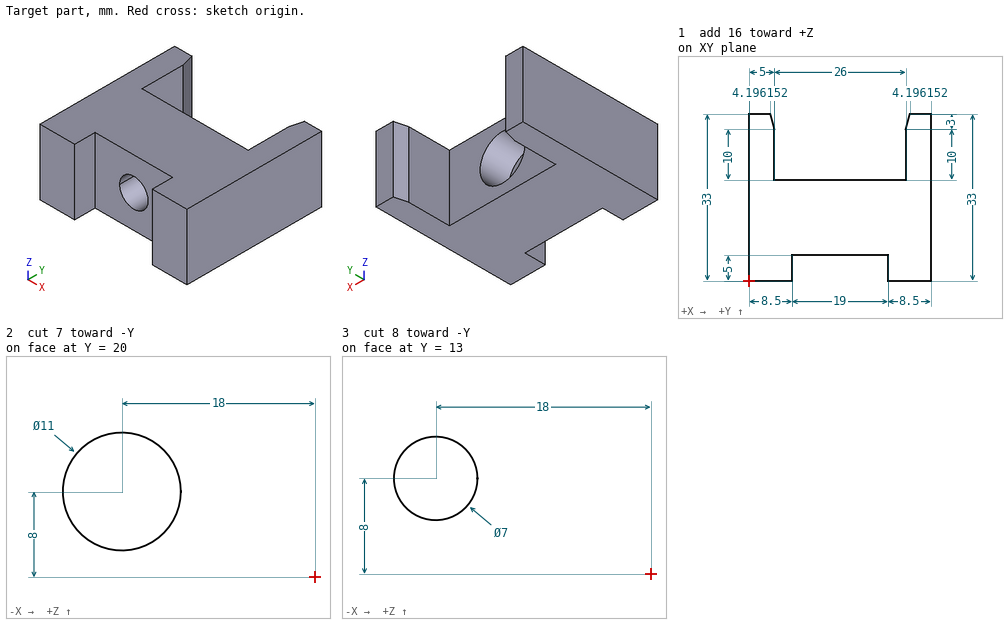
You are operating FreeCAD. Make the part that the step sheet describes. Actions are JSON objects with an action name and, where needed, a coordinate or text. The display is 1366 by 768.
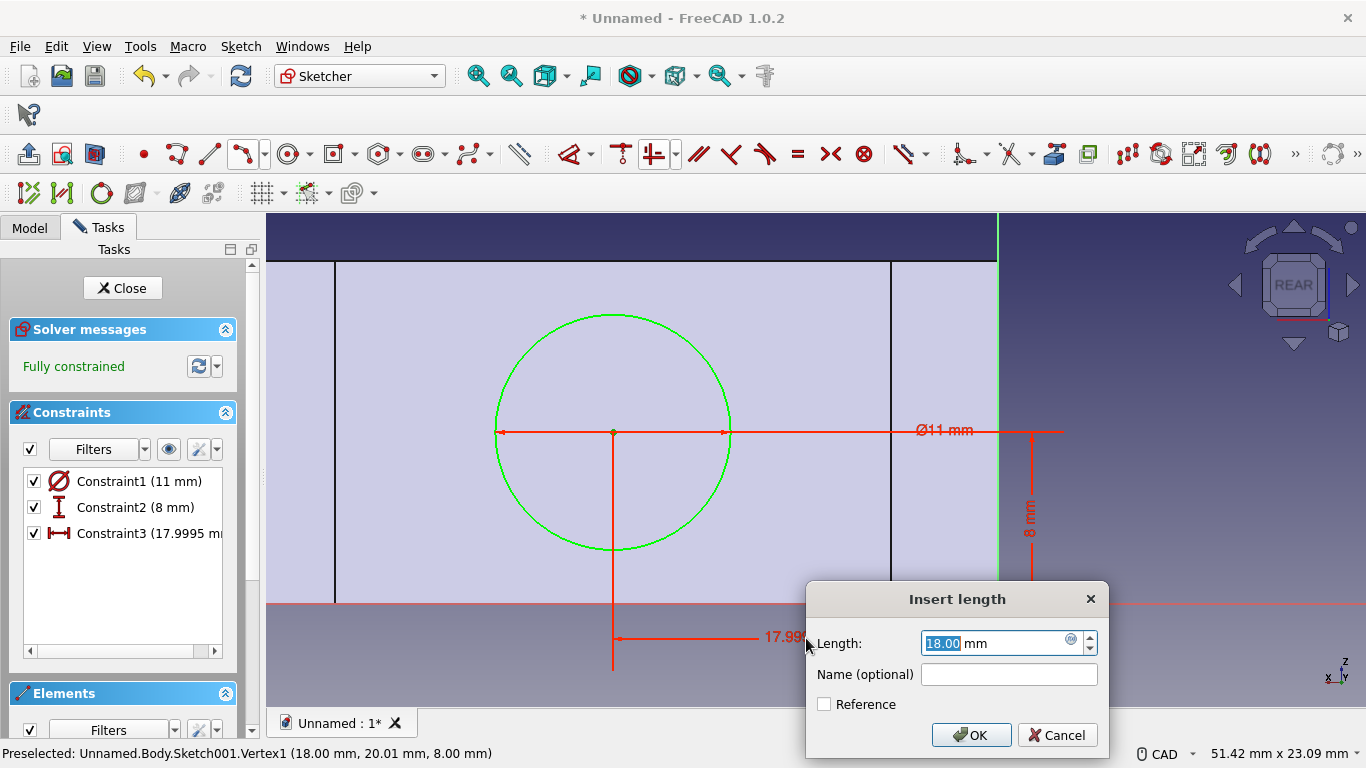
{"action": "type", "text": "18"}
{"action": "key", "text": "Return"}
{"action": "key", "text": "Escape"}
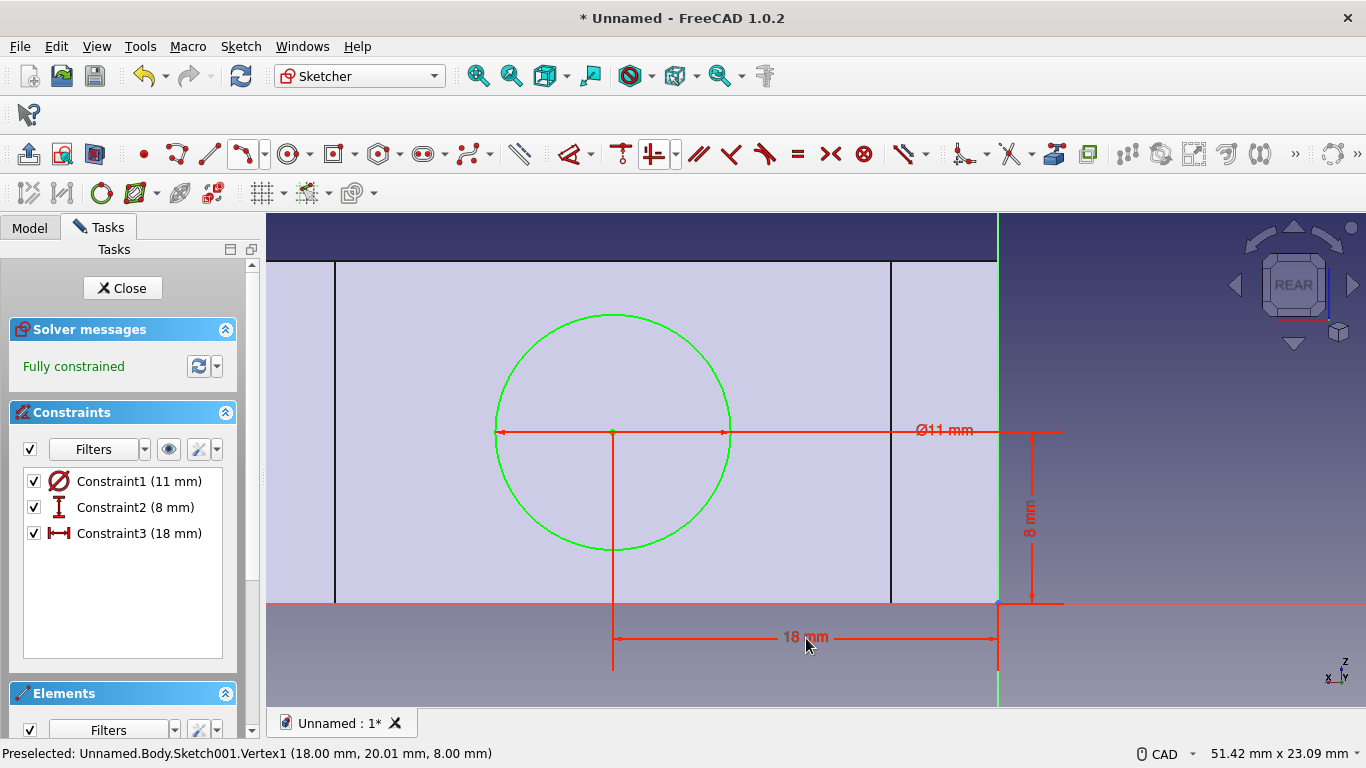
{"action": "left_click", "coordinate": [123, 288]}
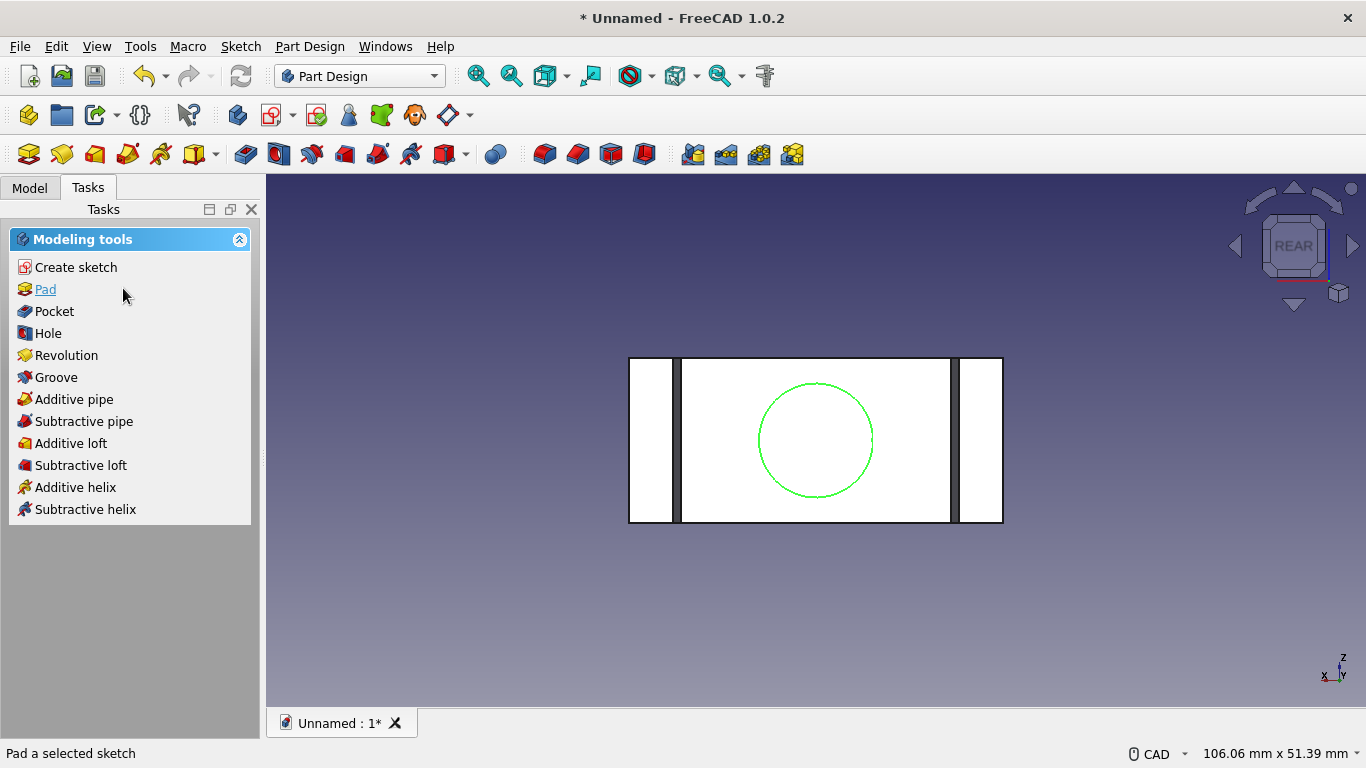
{"action": "left_click", "coordinate": [246, 154]}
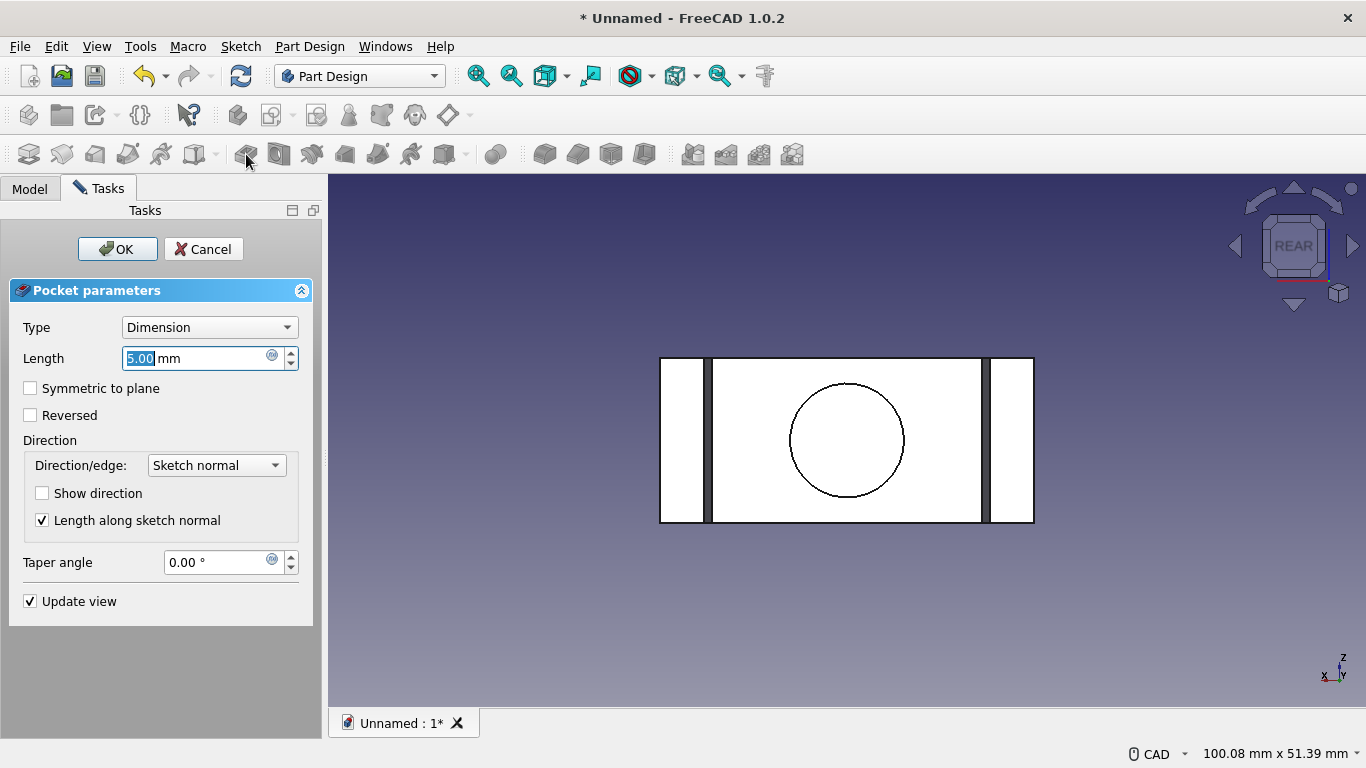
{"action": "type", "text": "7"}
{"action": "key", "text": "Tab"}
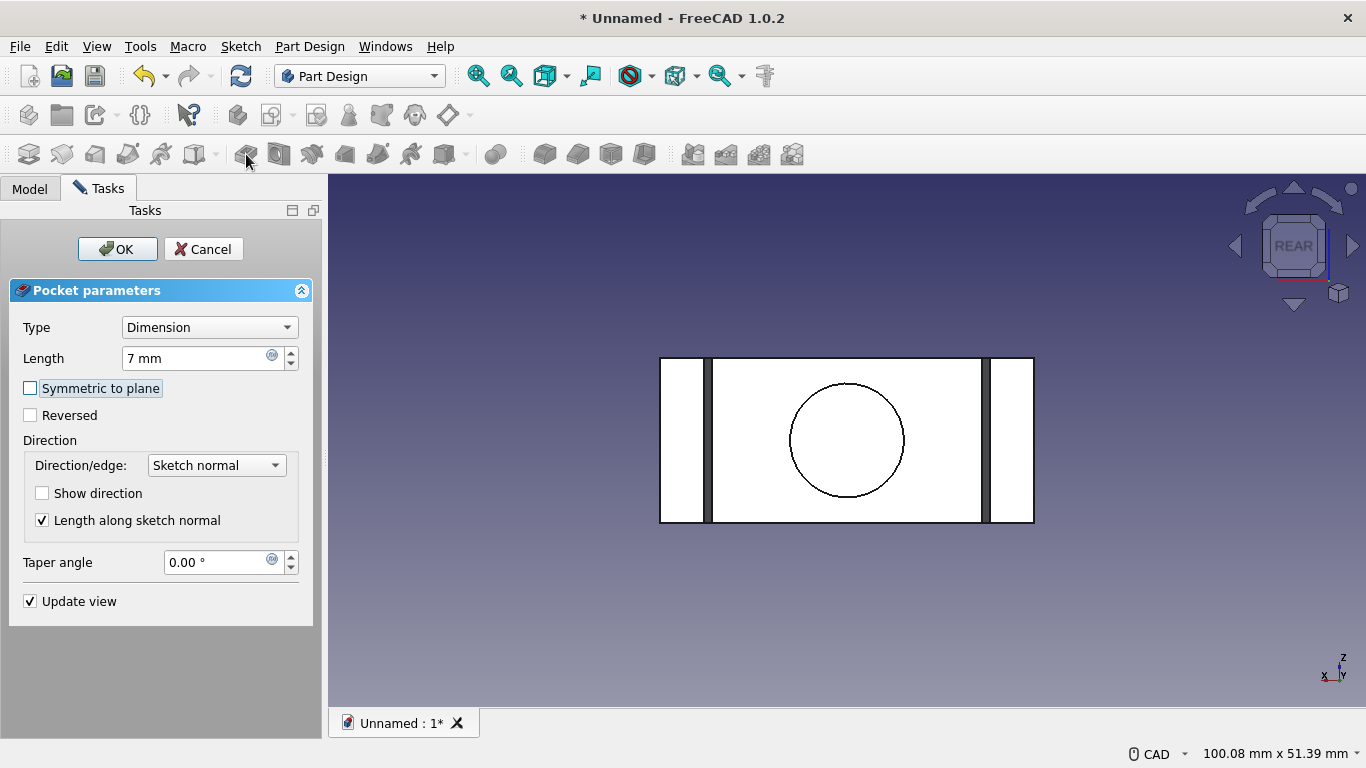
{"action": "left_click", "coordinate": [118, 249]}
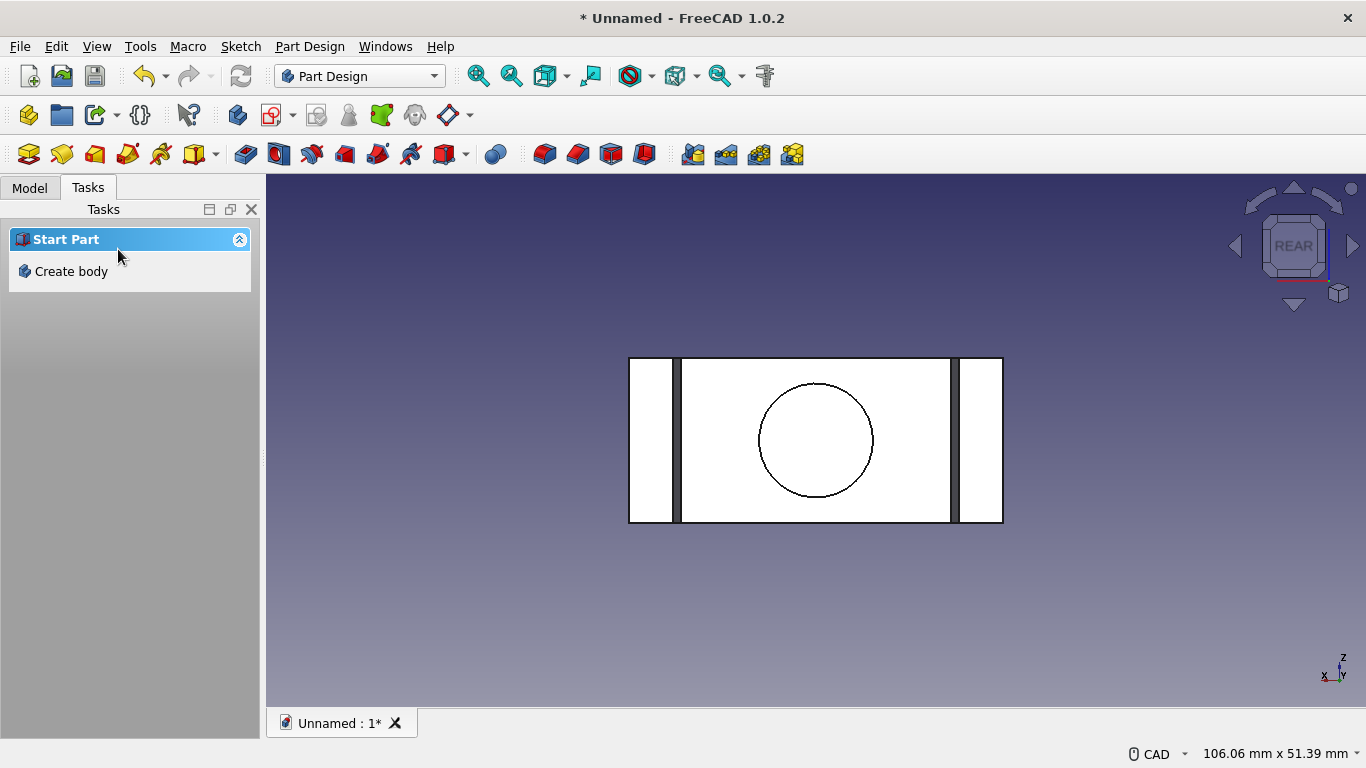
{"action": "left_click", "coordinate": [479, 76]}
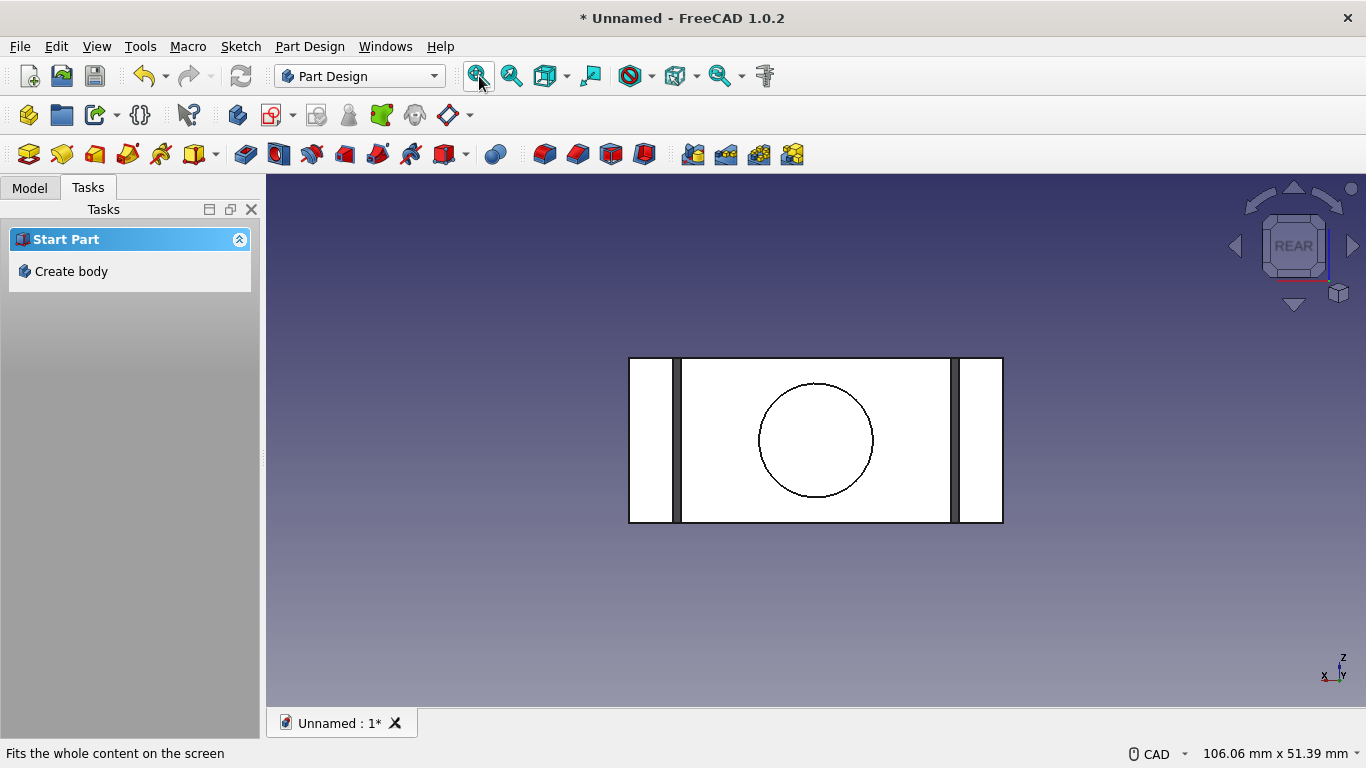
{"action": "left_click", "coordinate": [816, 439]}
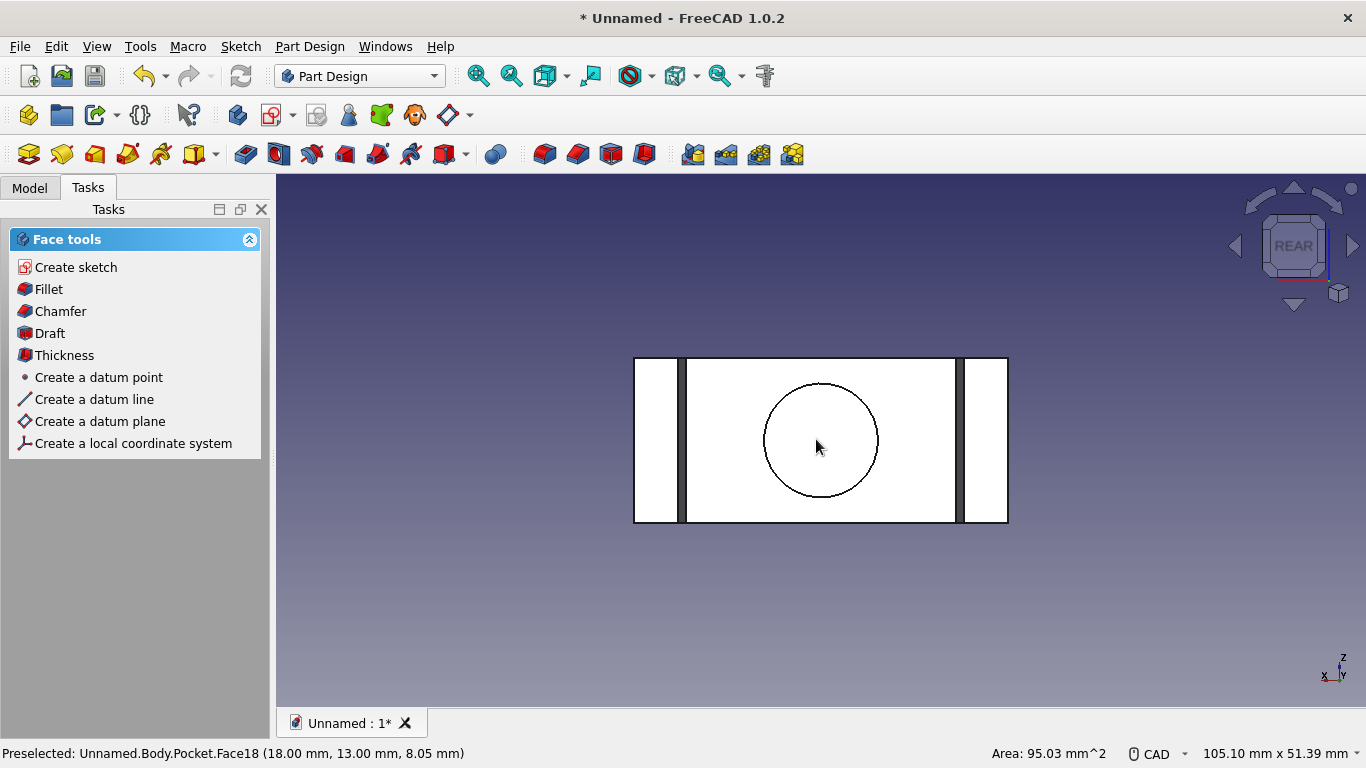
{"action": "left_click", "coordinate": [270, 116]}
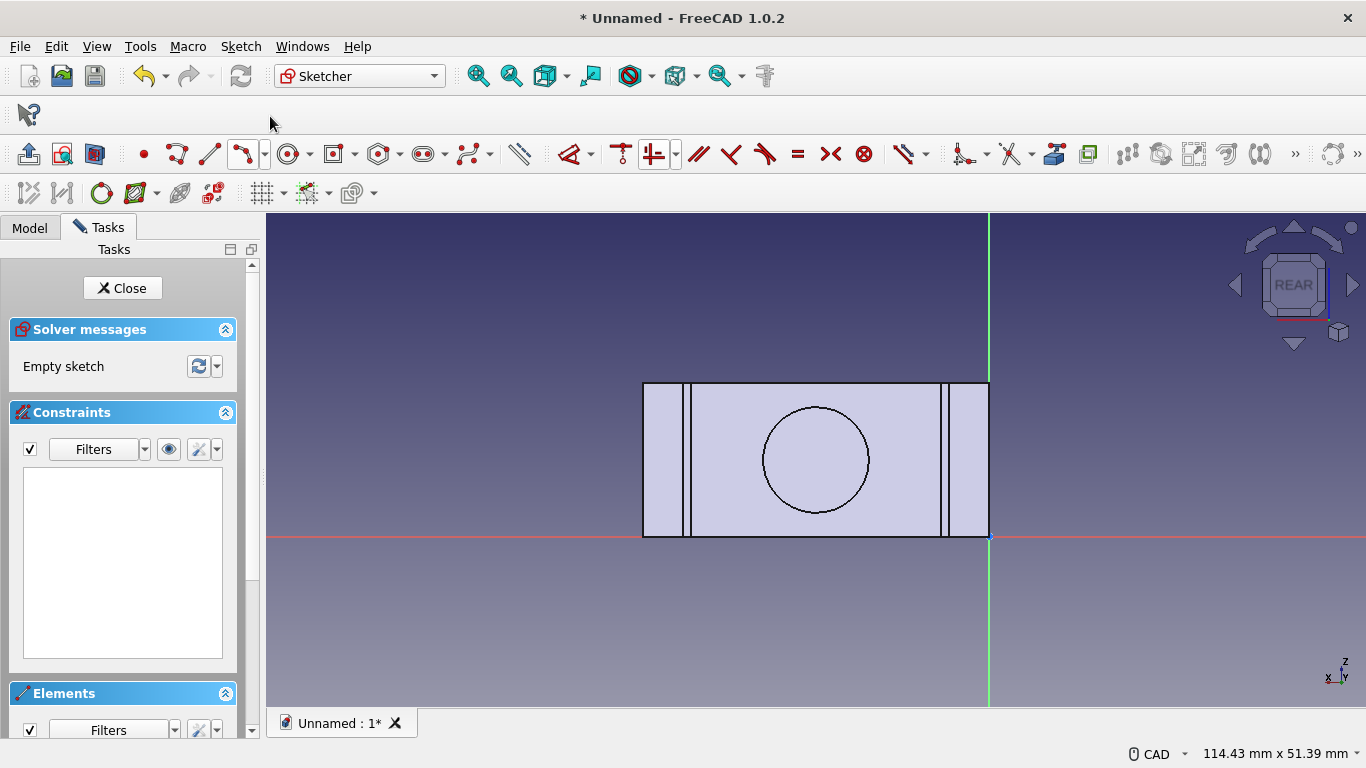
{"action": "scroll", "coordinate": [833, 460], "scroll_direction": "up", "scroll_amount": 8}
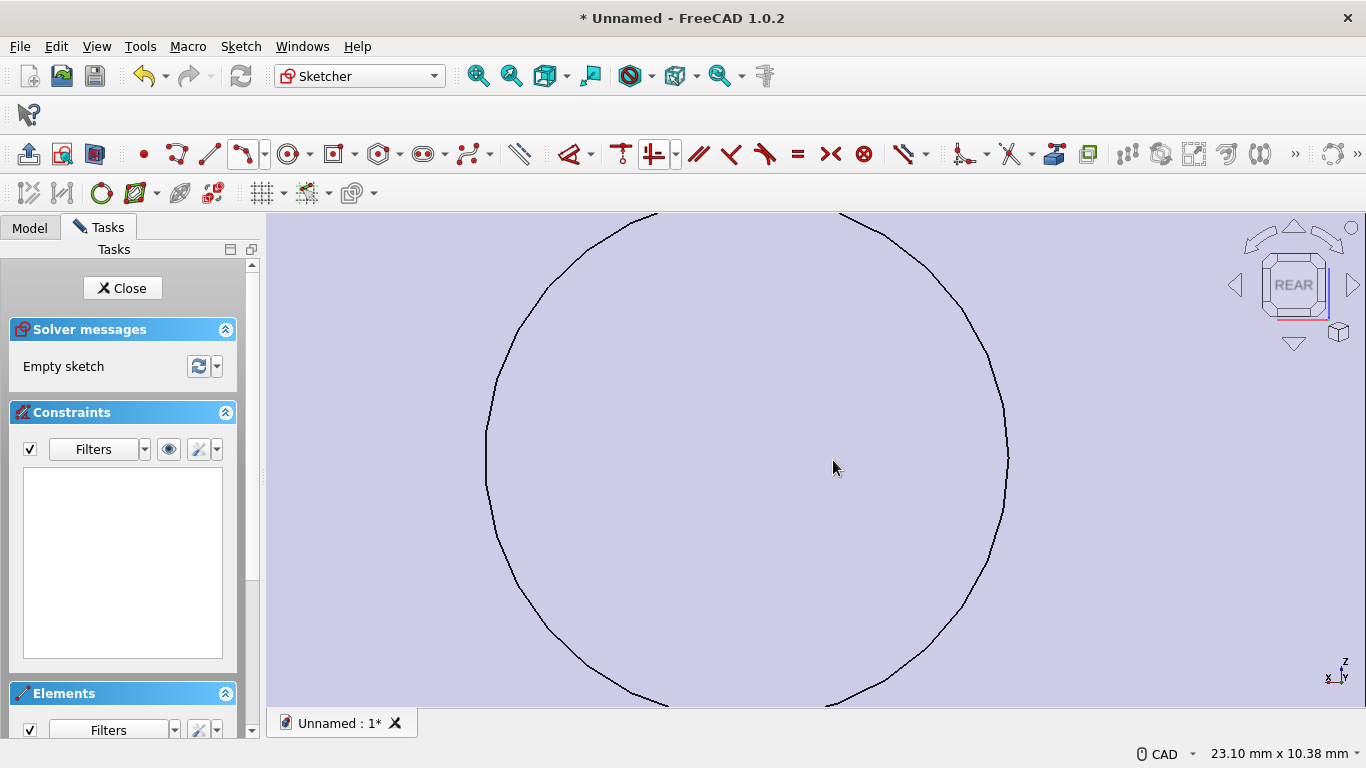
{"action": "left_click", "coordinate": [288, 154]}